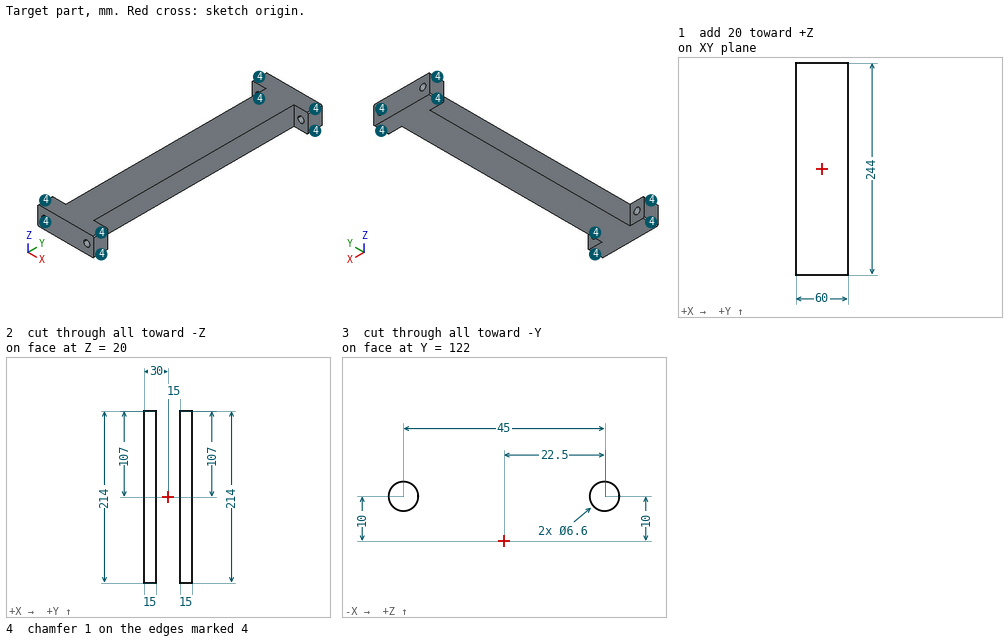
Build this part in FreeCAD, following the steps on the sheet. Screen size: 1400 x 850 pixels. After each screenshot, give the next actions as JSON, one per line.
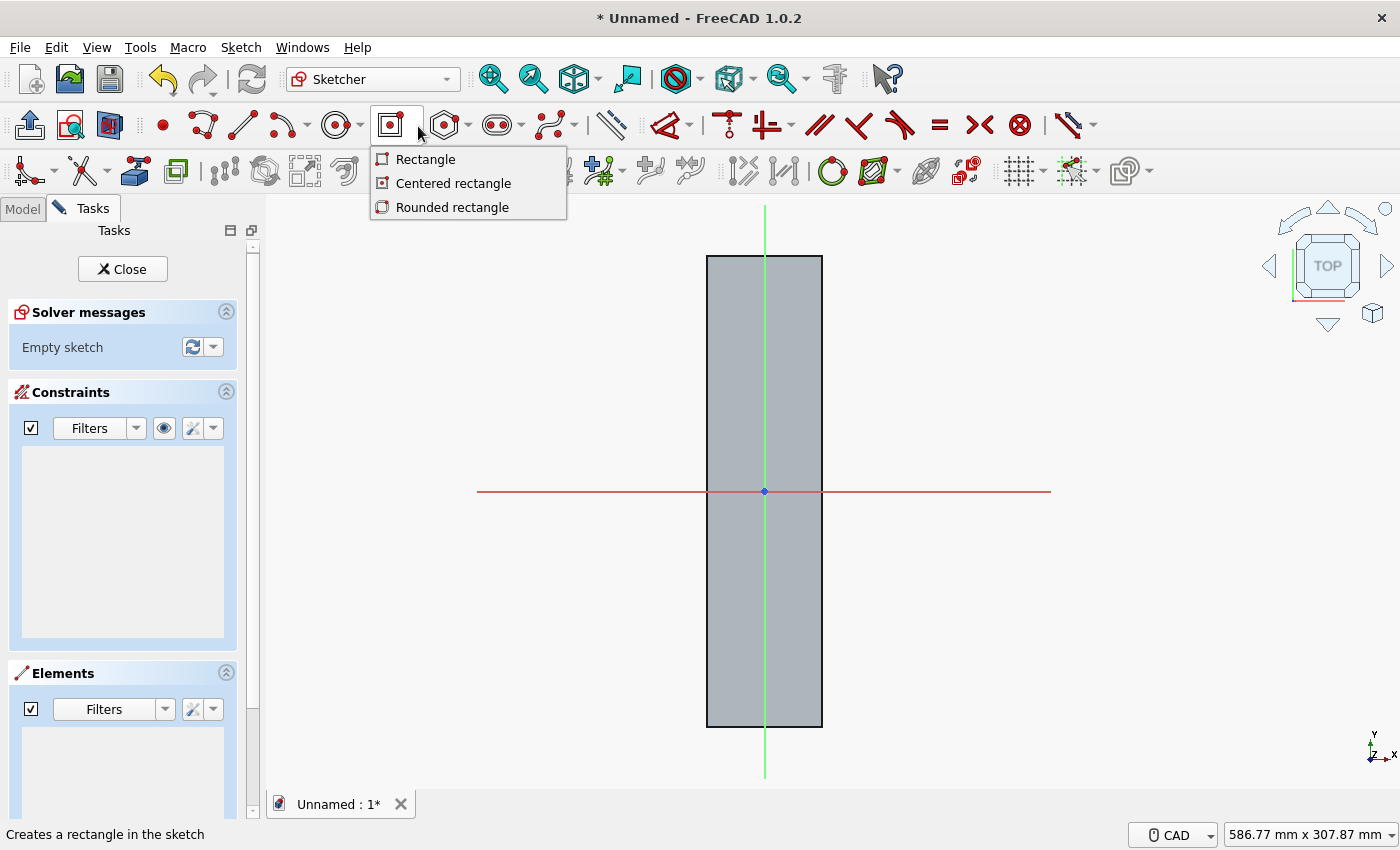
{"action": "left_click", "coordinate": [468, 159]}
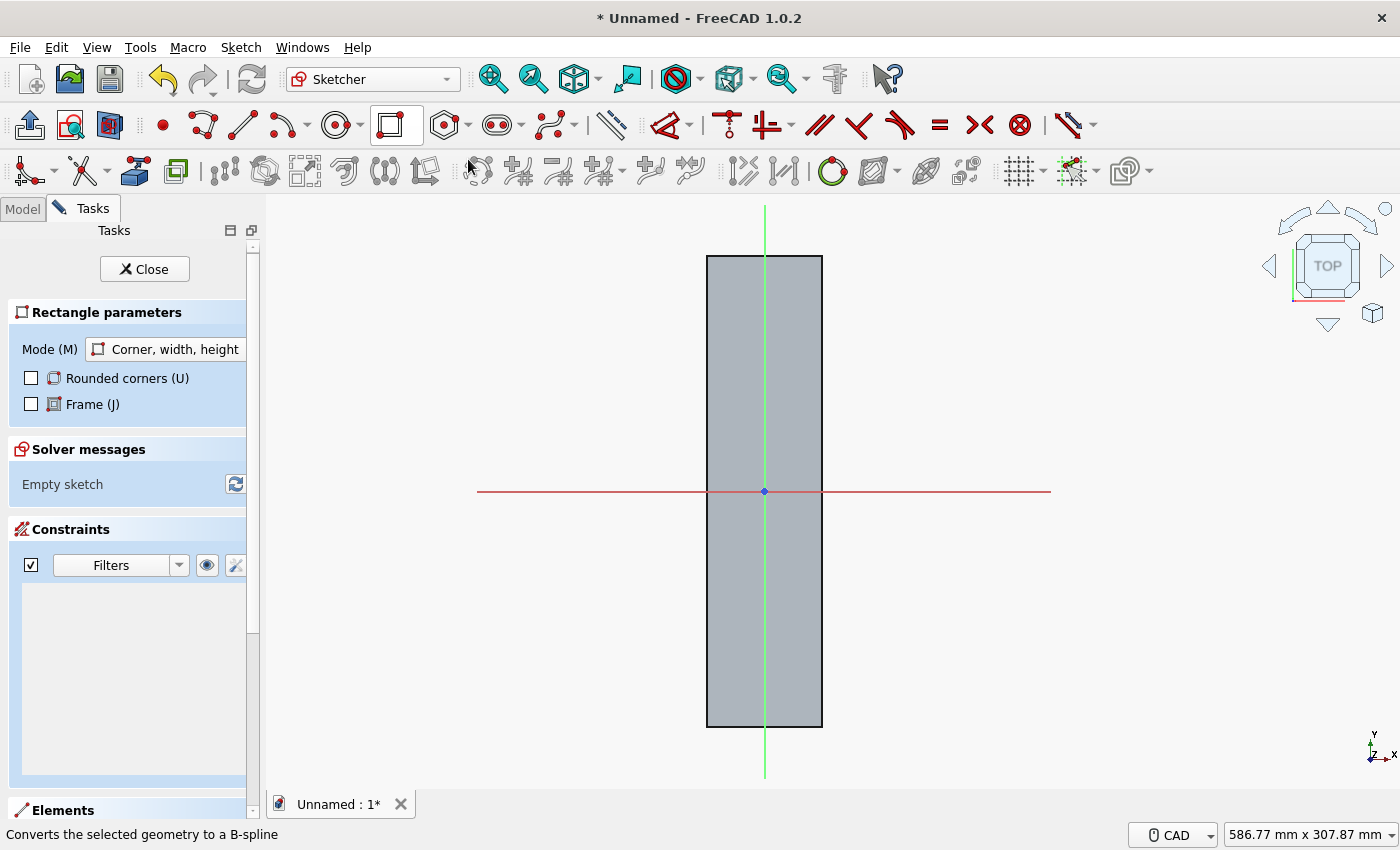
{"action": "left_click", "coordinate": [707, 285]}
{"action": "mouse_move", "coordinate": [736, 698]}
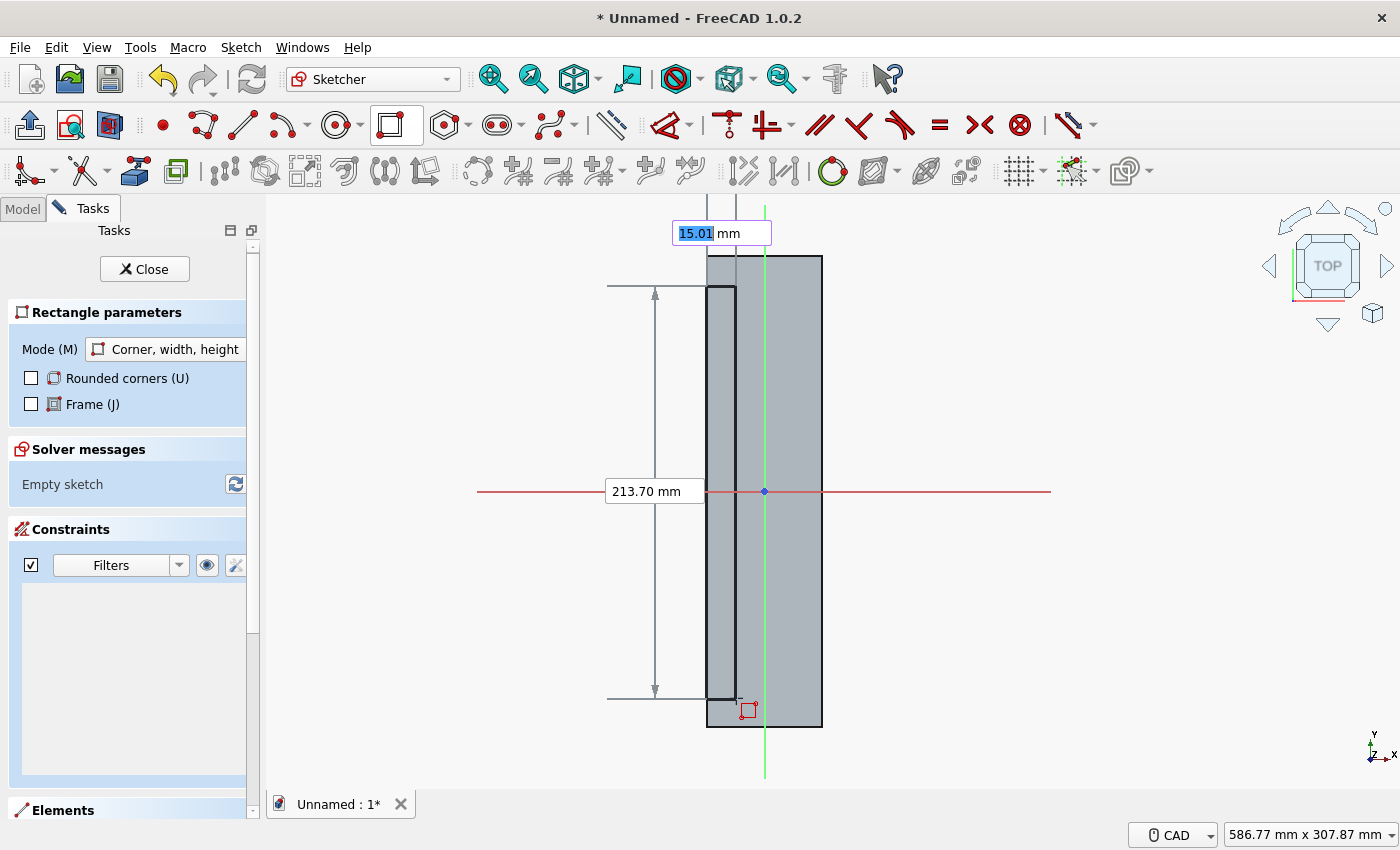
{"action": "type", "text": "15"}
{"action": "key", "text": "Tab"}
{"action": "type", "text": "214"}
{"action": "key", "text": "Return"}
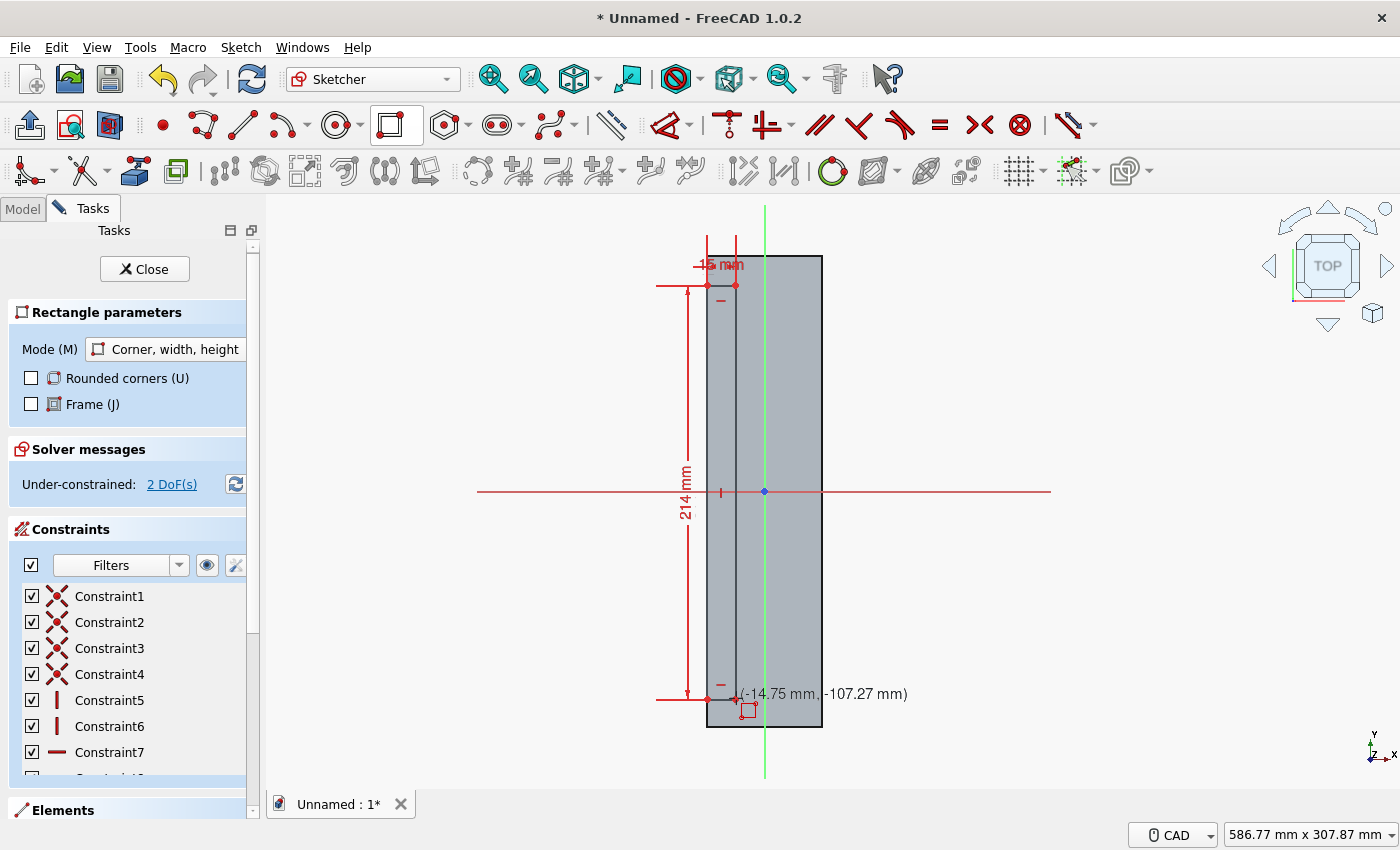
{"action": "left_click", "coordinate": [793, 285]}
{"action": "mouse_move", "coordinate": [822, 698]}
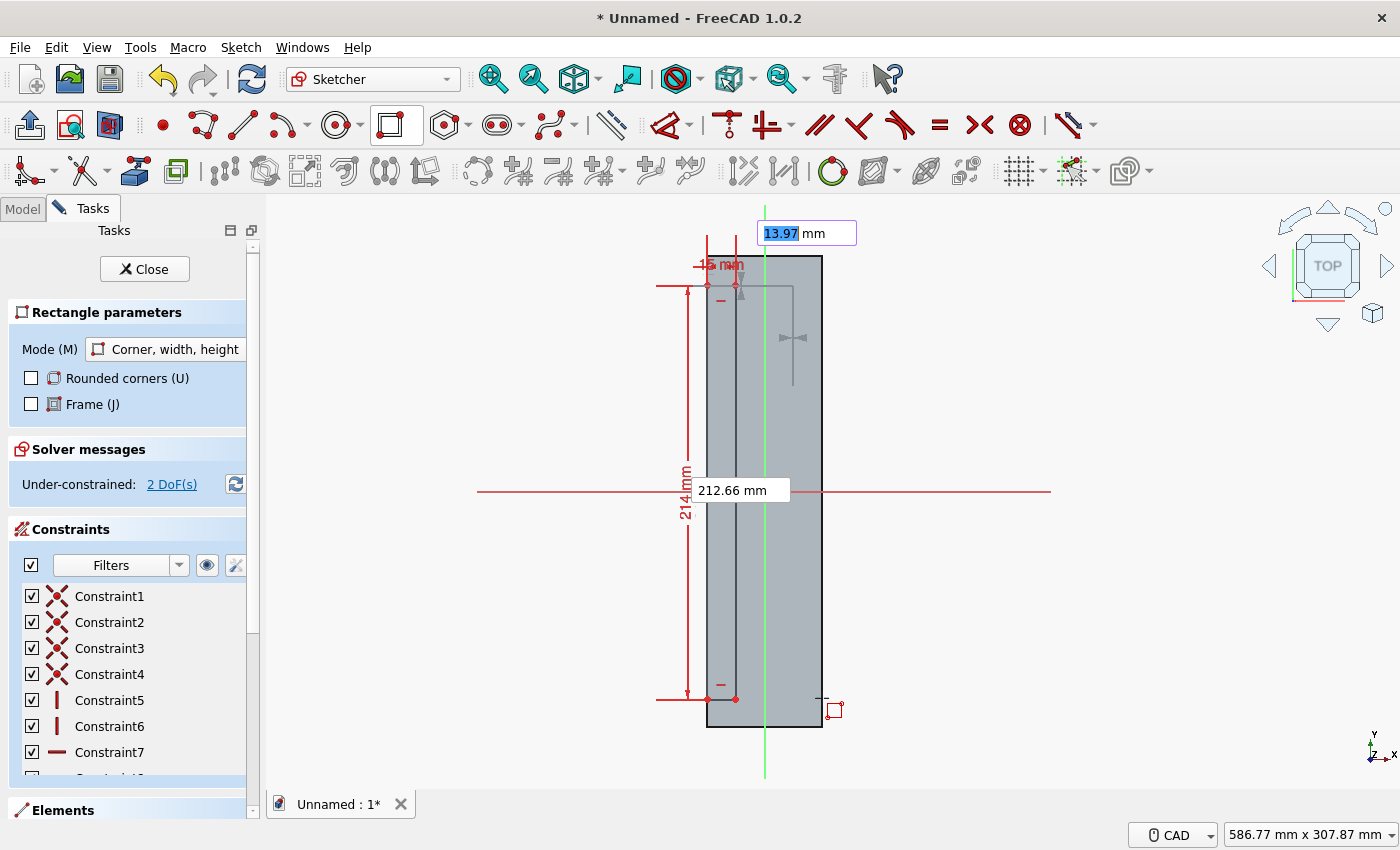
{"action": "type", "text": "15"}
{"action": "key", "text": "Tab"}
{"action": "type", "text": "214"}
{"action": "key", "text": "Return"}
{"action": "key", "text": "Escape"}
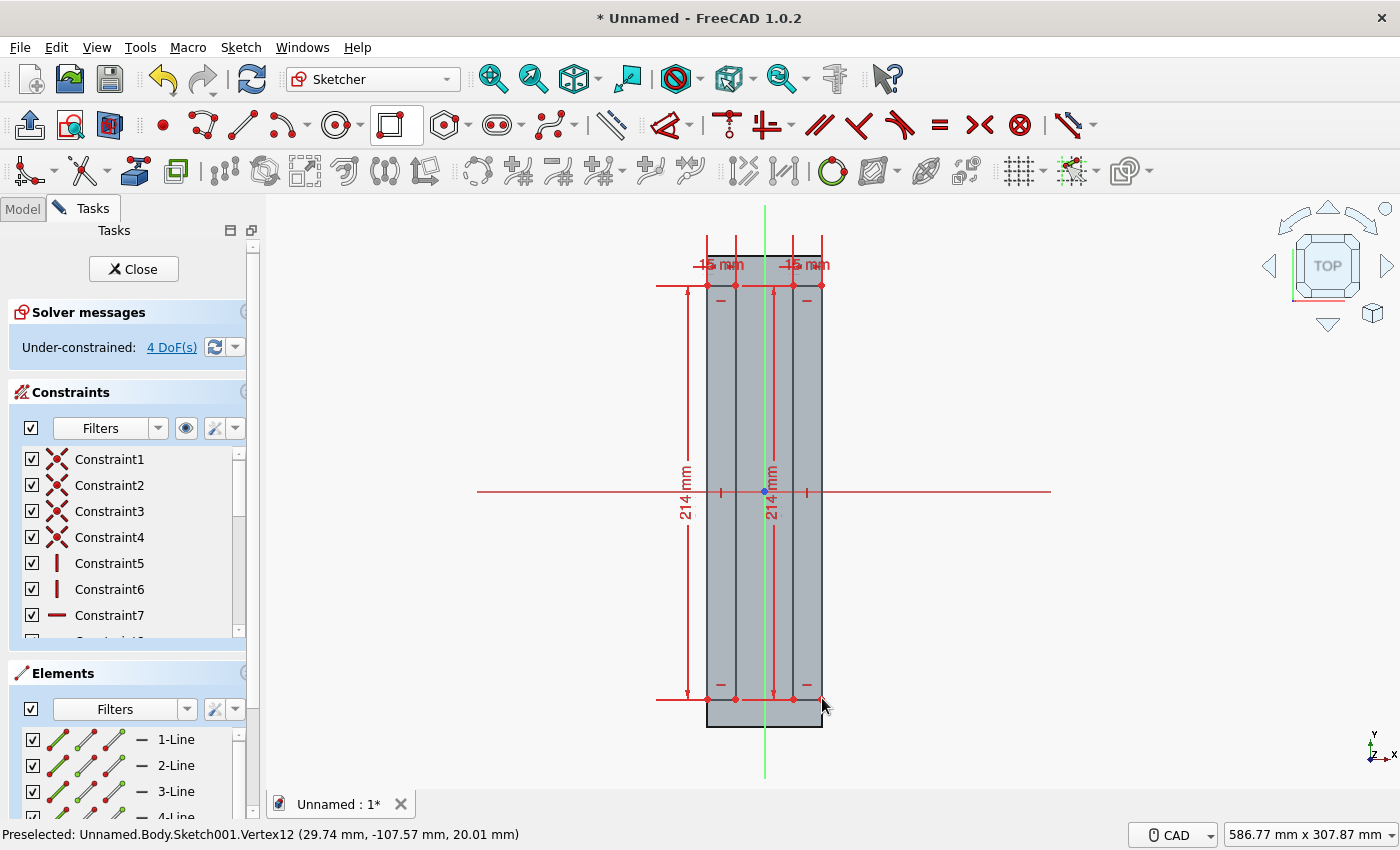
{"action": "left_click", "coordinate": [666, 126]}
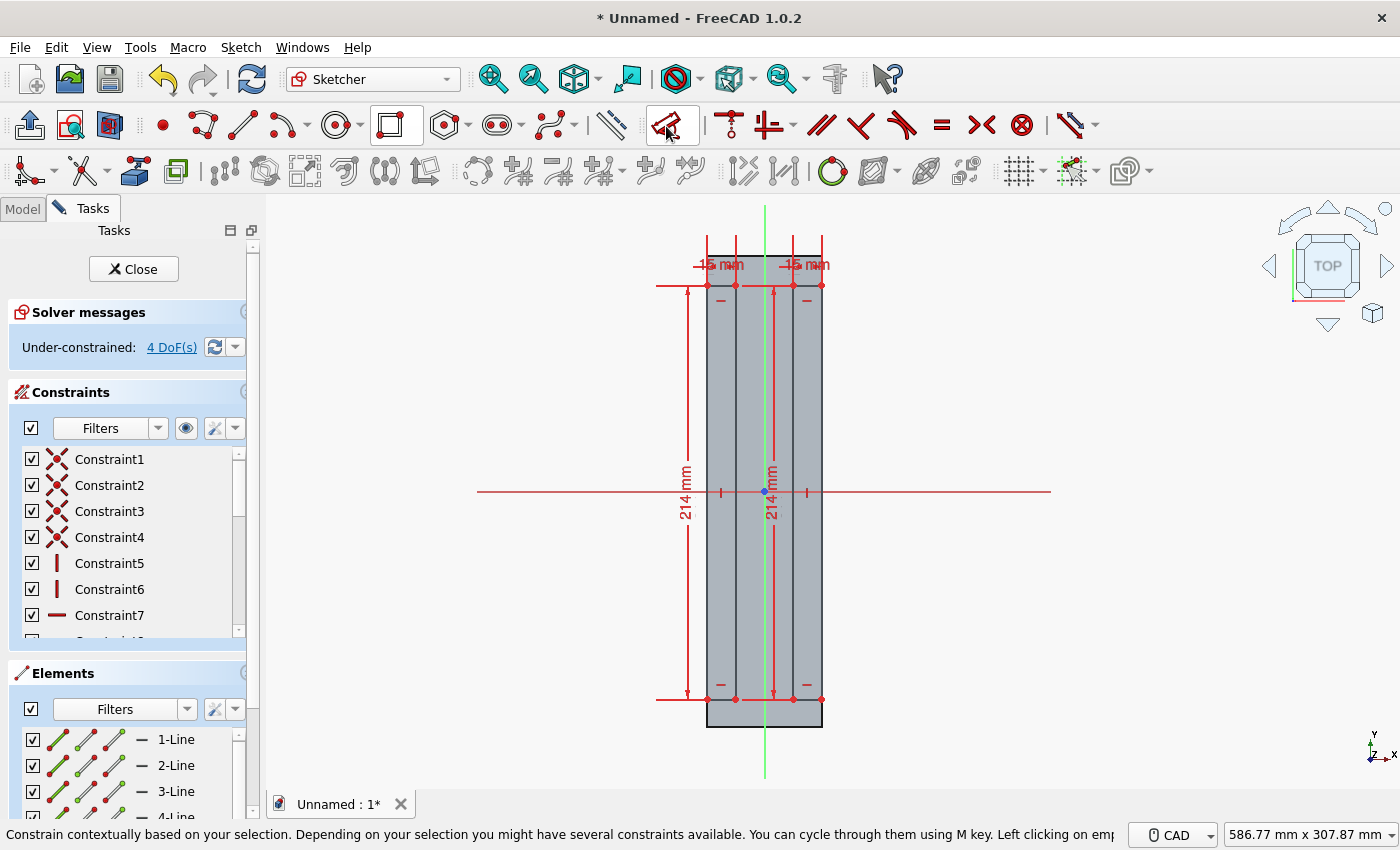
{"action": "left_click", "coordinate": [707, 286]}
{"action": "left_click", "coordinate": [736, 252]}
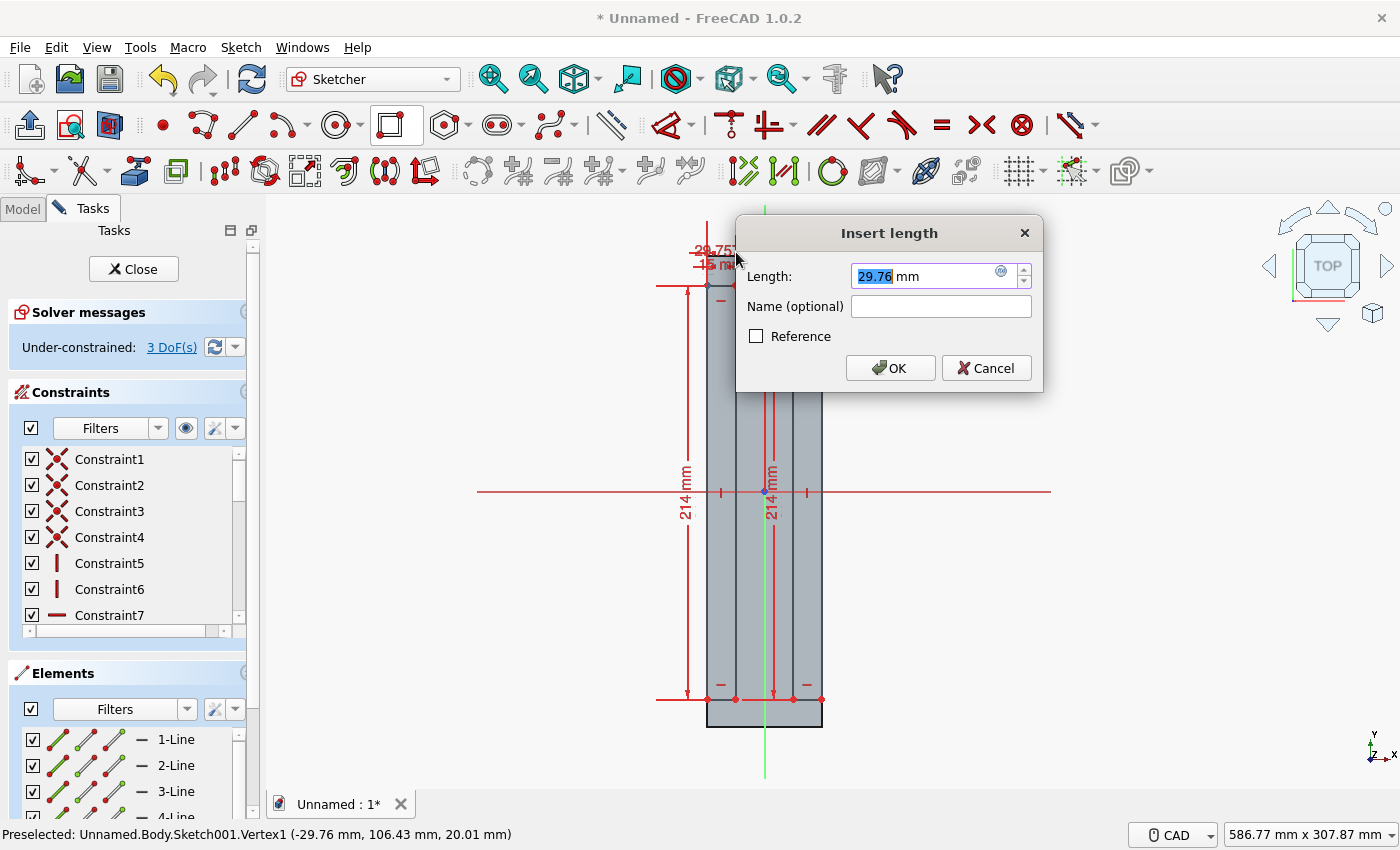
{"action": "type", "text": "30"}
{"action": "key", "text": "Return"}